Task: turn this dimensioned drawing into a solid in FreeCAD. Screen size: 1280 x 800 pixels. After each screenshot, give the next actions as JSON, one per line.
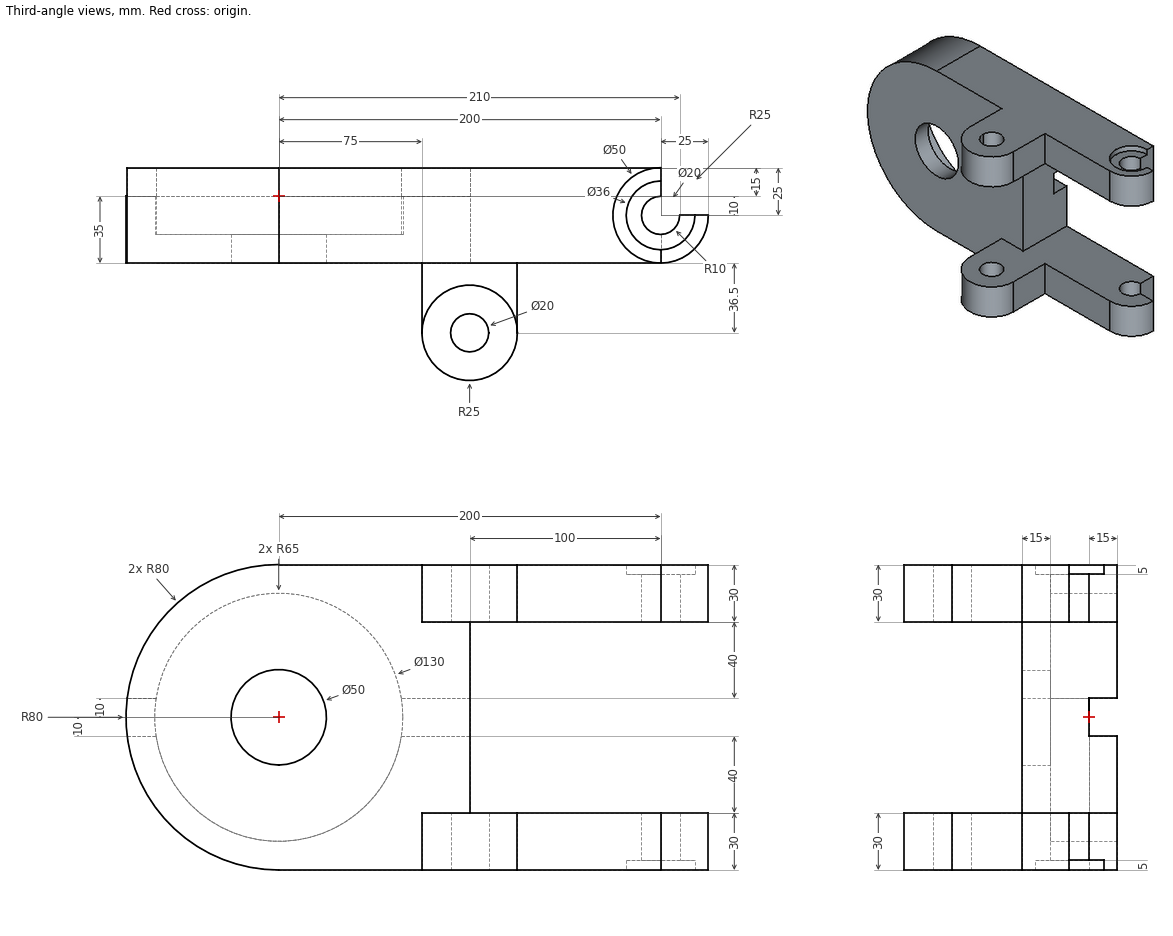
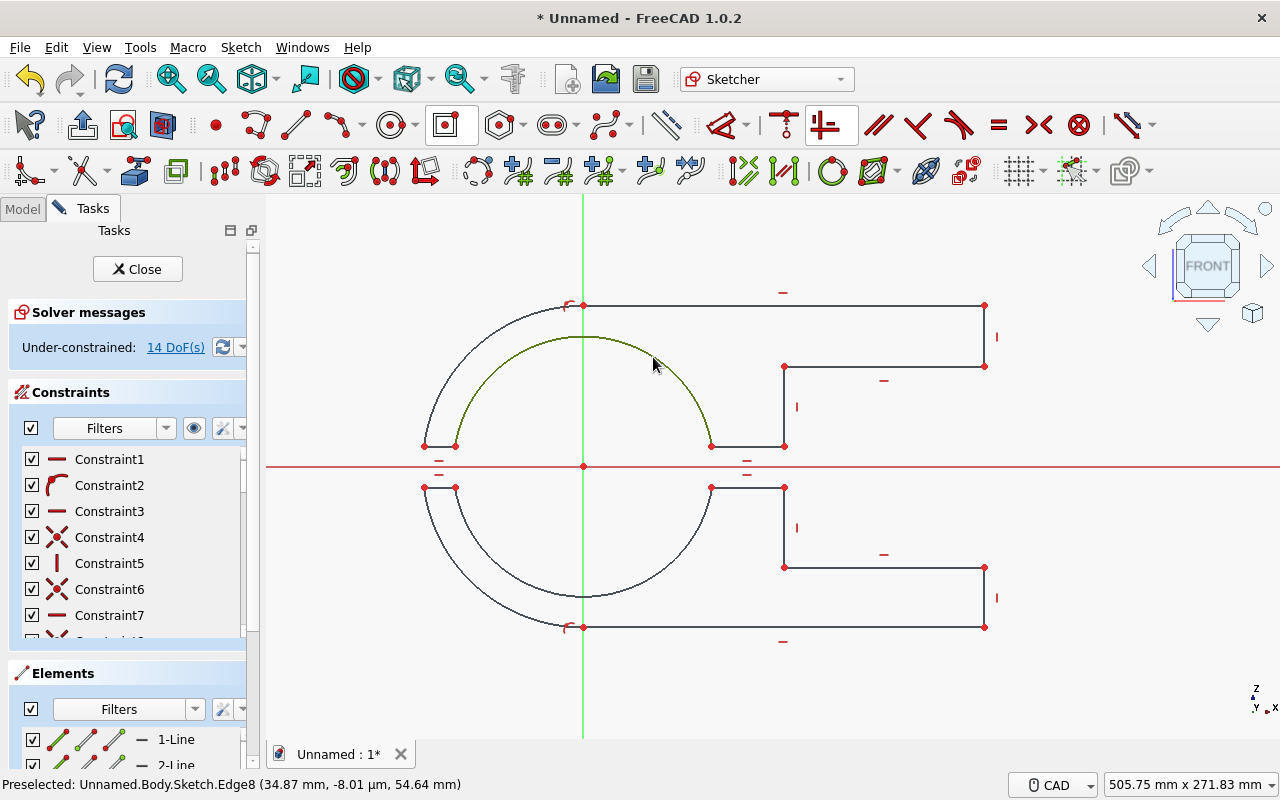
{"action": "left_click", "coordinate": [514, 577]}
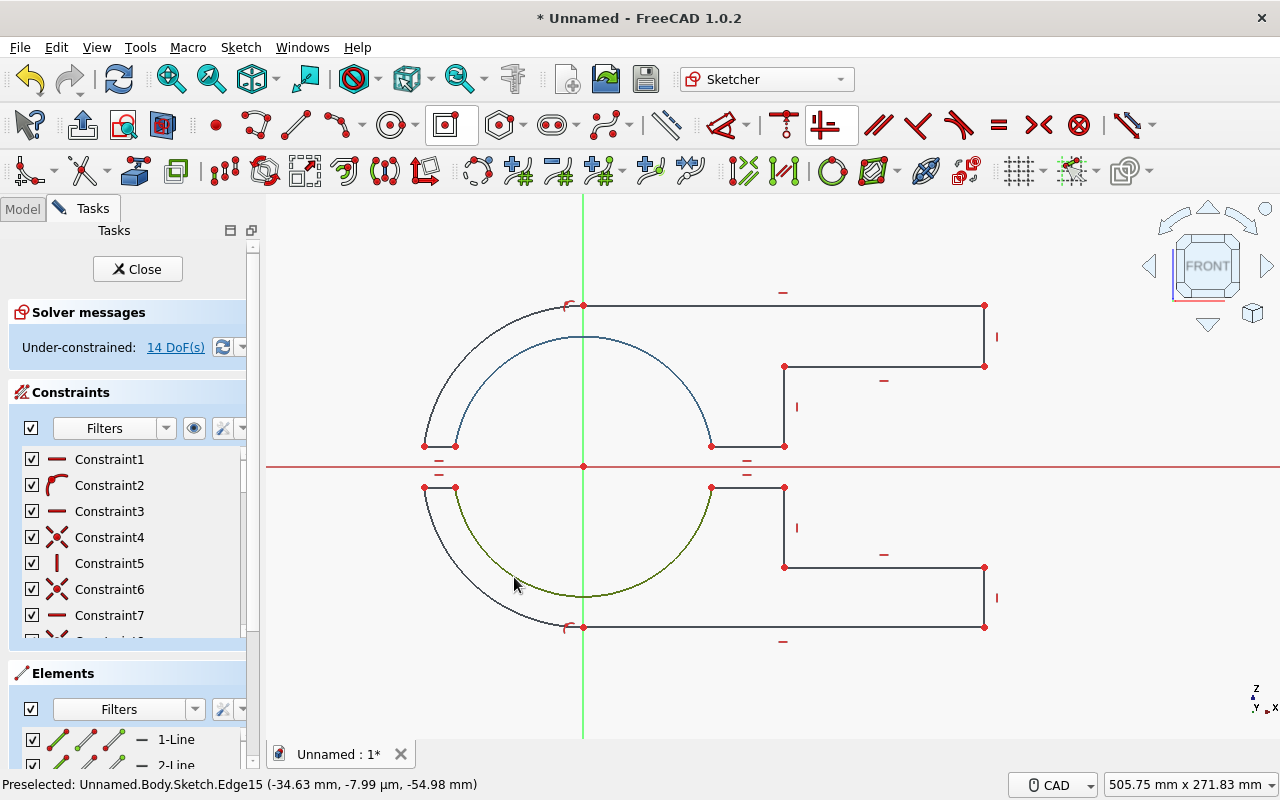
{"action": "left_click", "coordinate": [1000, 126]}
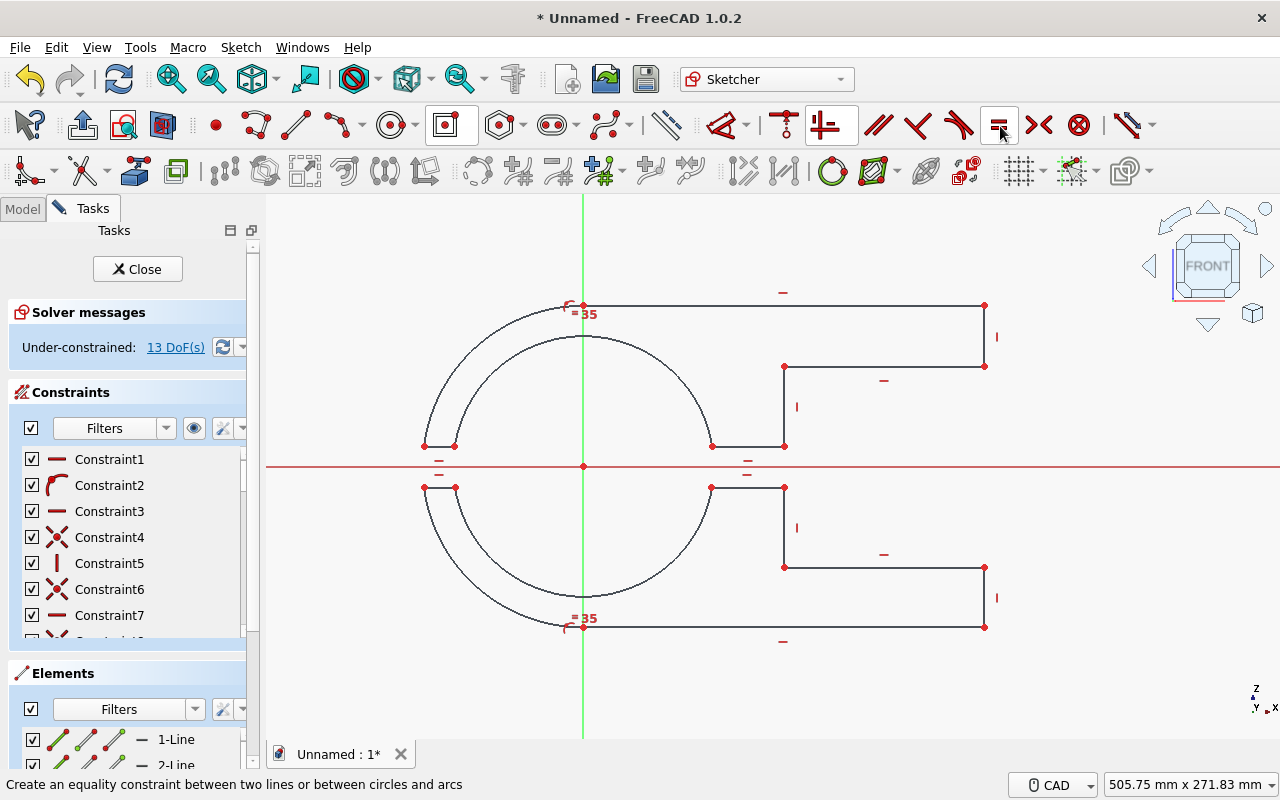
{"action": "left_click", "coordinate": [516, 321]}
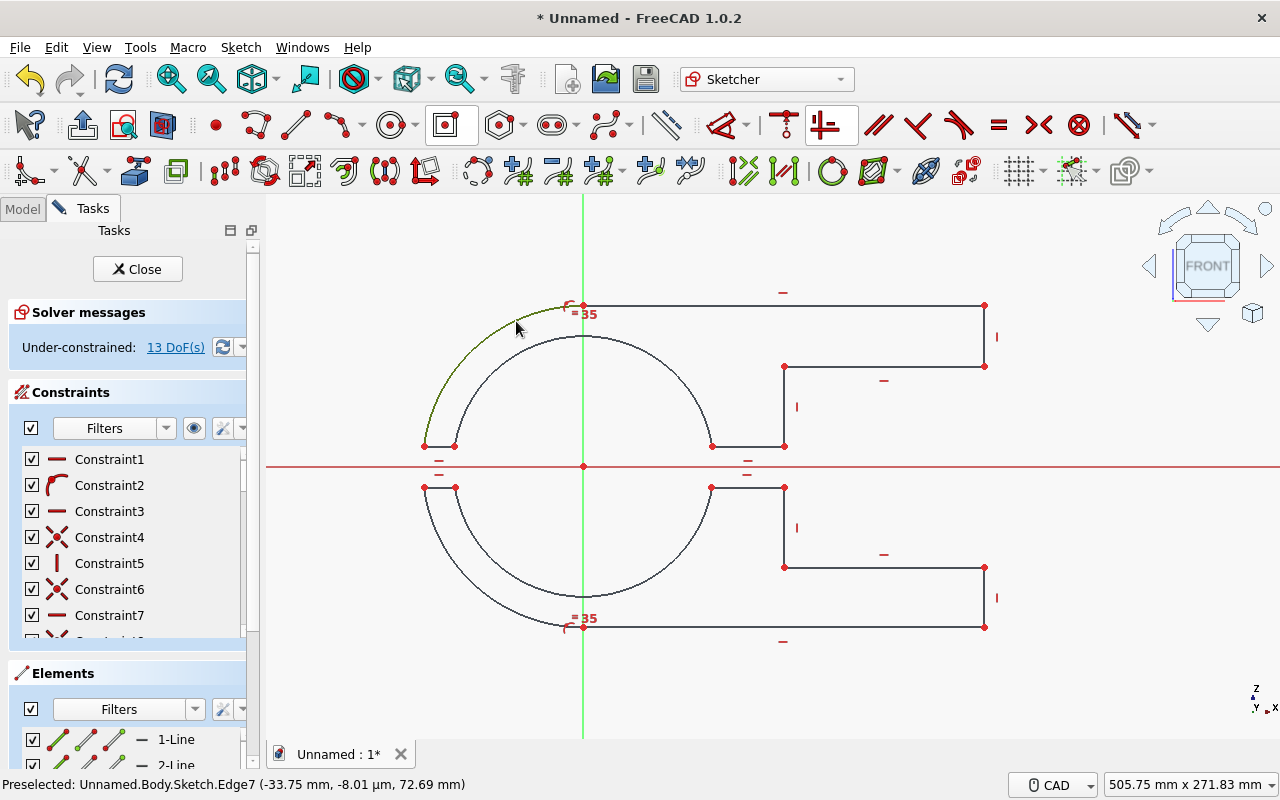
{"action": "left_click", "coordinate": [448, 553]}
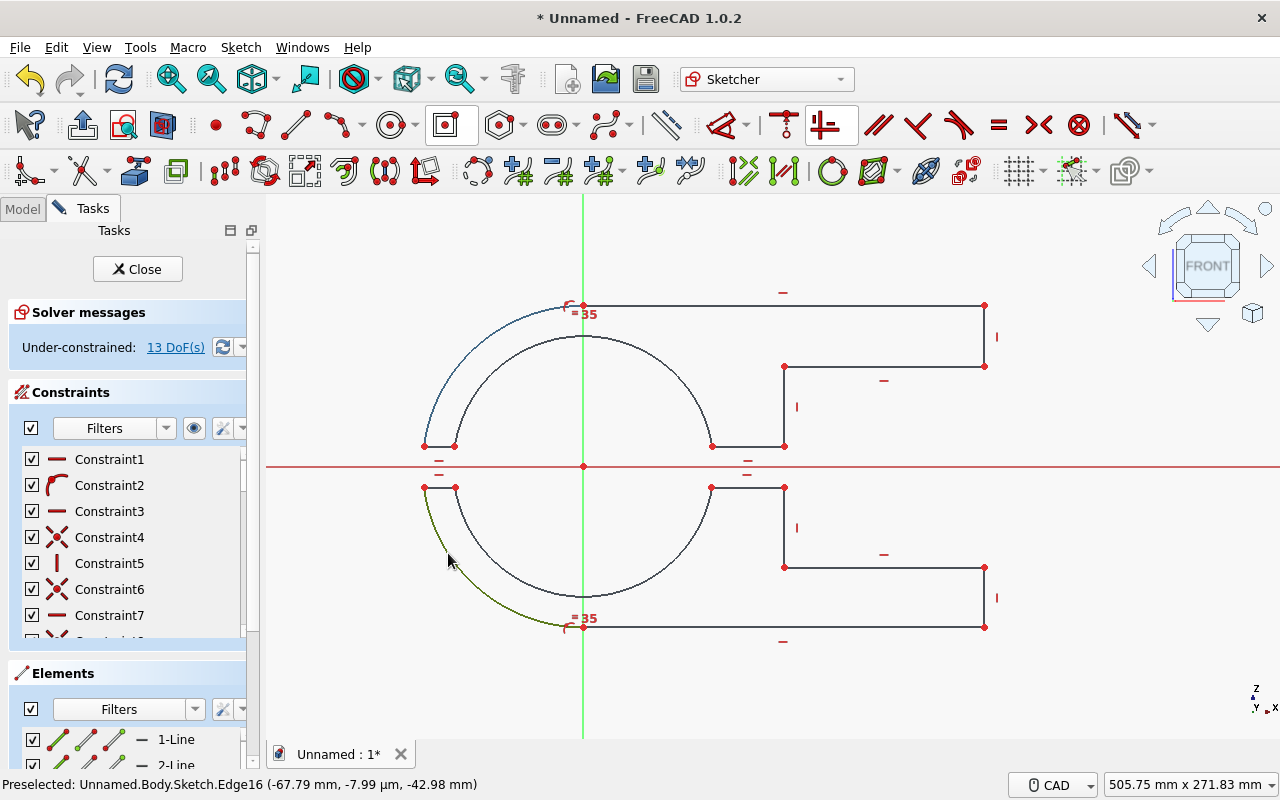
{"action": "key", "text": "e"}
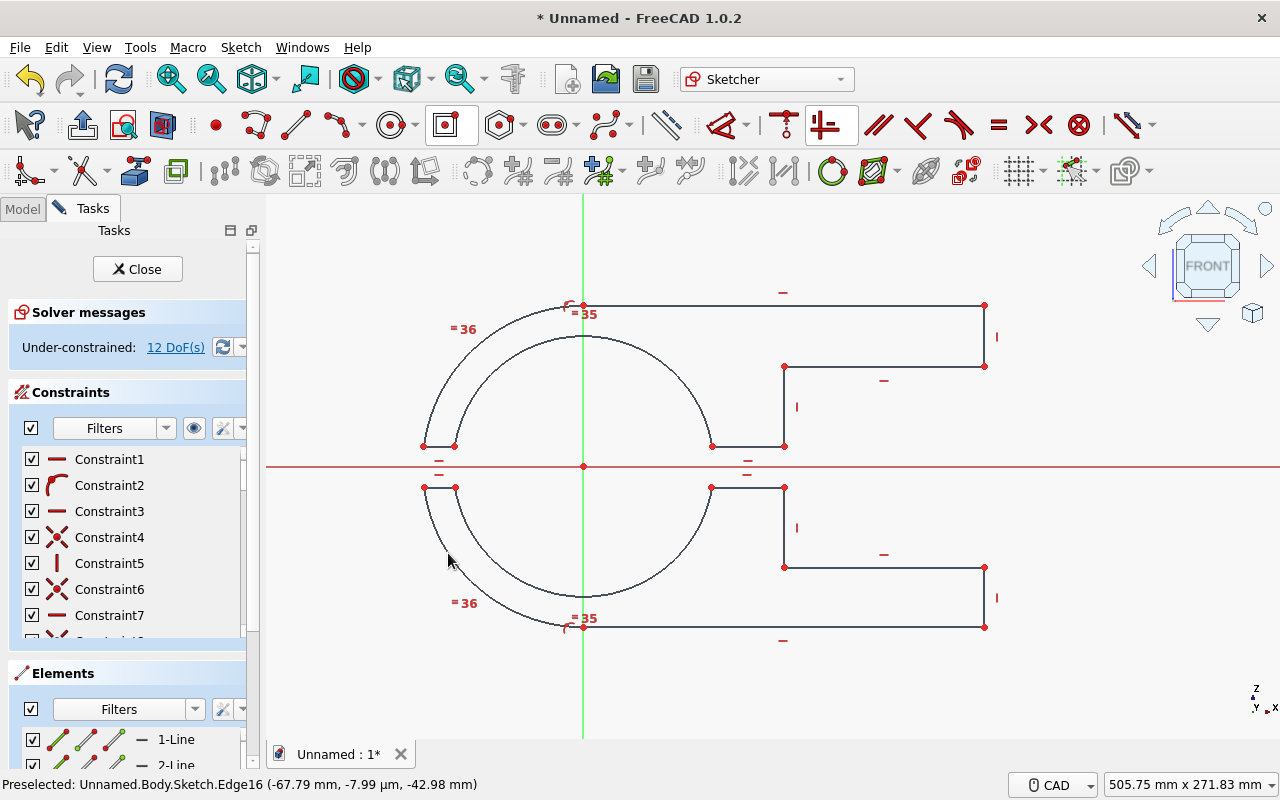
{"action": "left_click", "coordinate": [722, 126]}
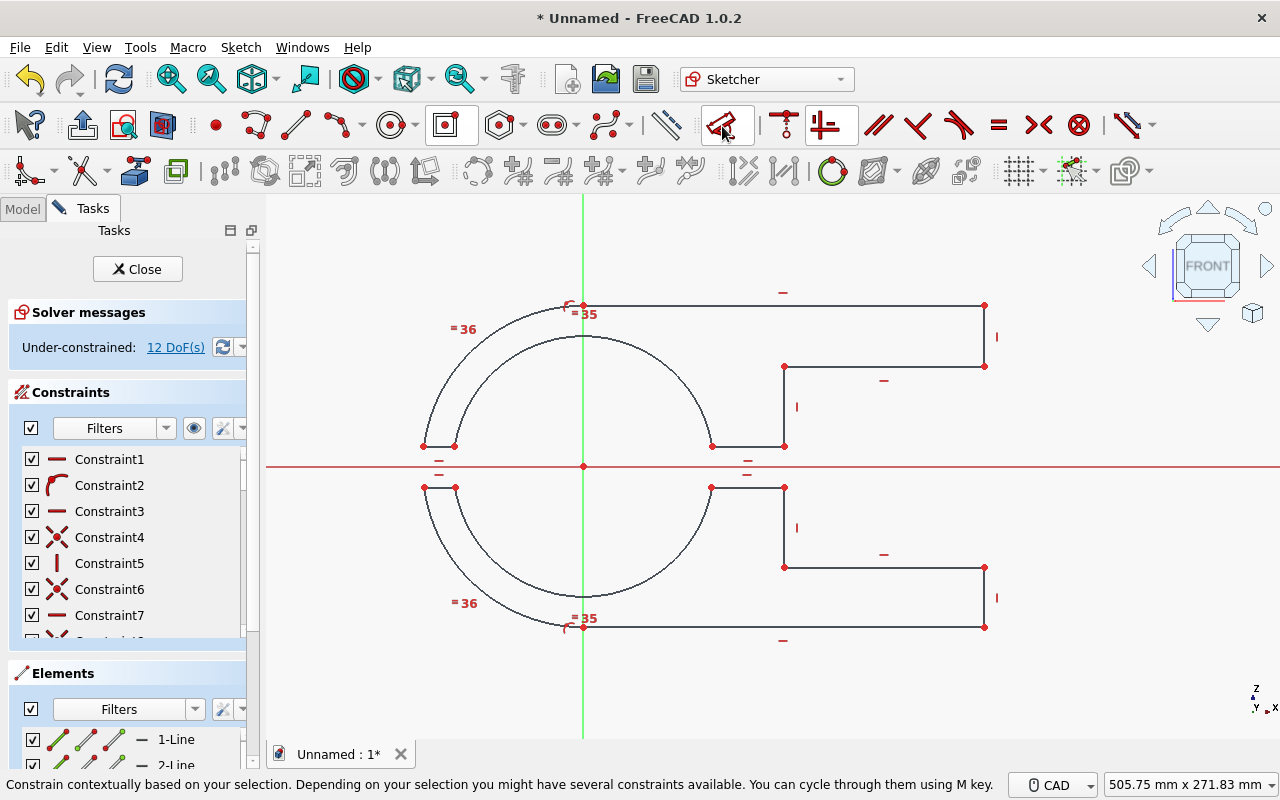
{"action": "left_click", "coordinate": [516, 321]}
{"action": "left_click", "coordinate": [503, 292]}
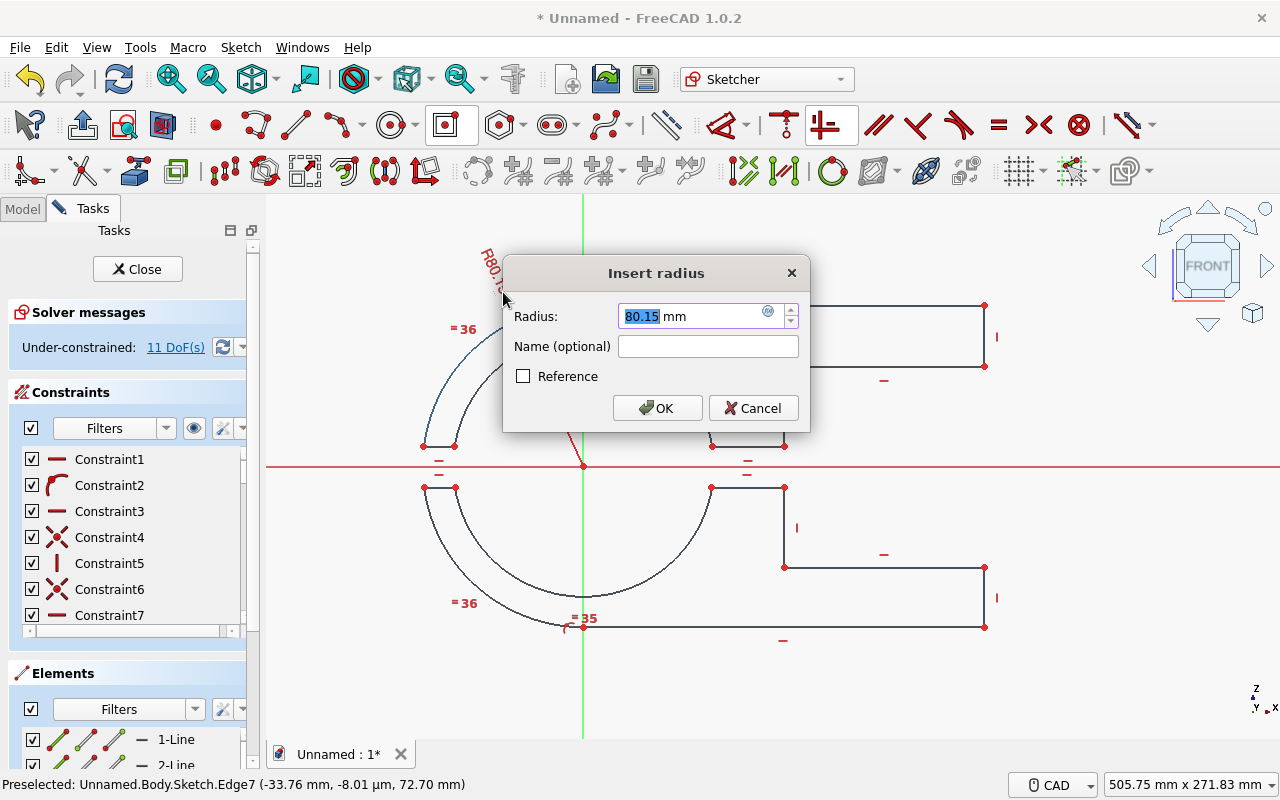
{"action": "type", "text": "80"}
{"action": "key", "text": "Return"}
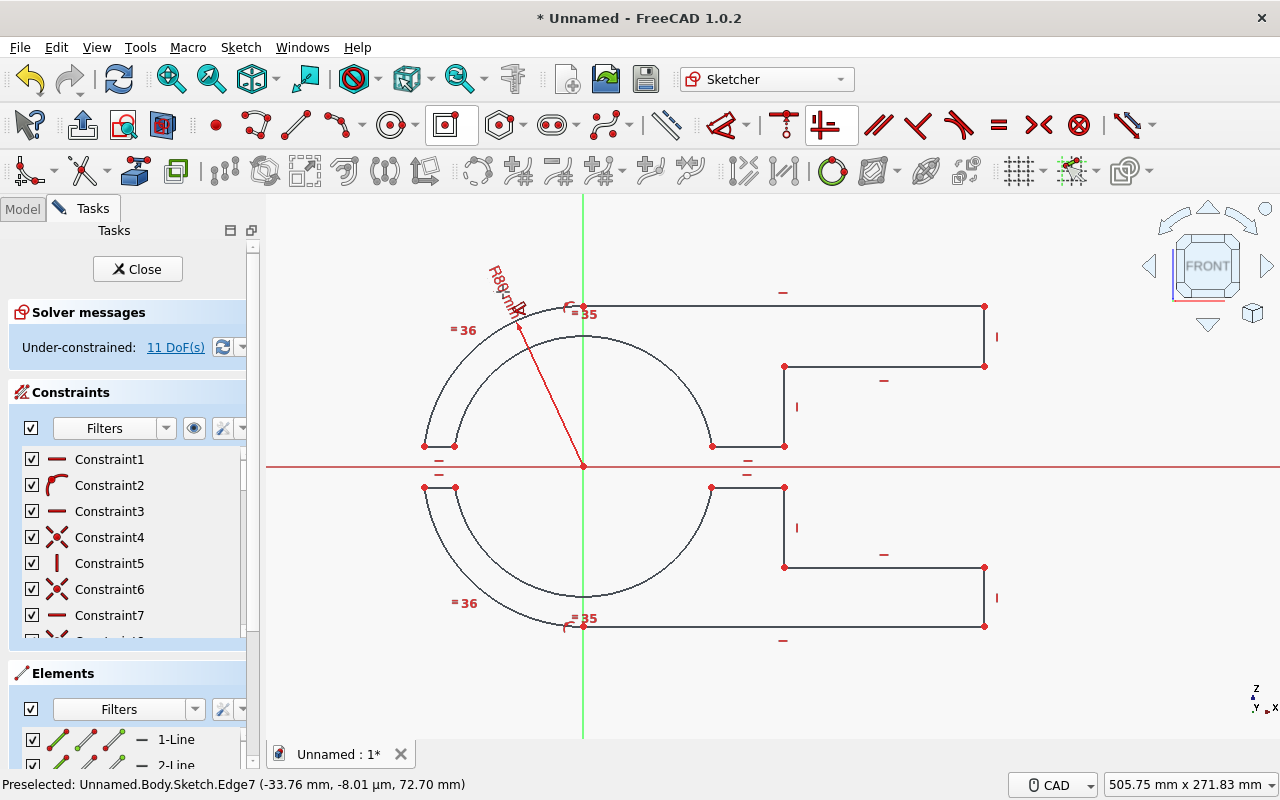
{"action": "left_click", "coordinate": [654, 357]}
{"action": "left_click", "coordinate": [671, 330]}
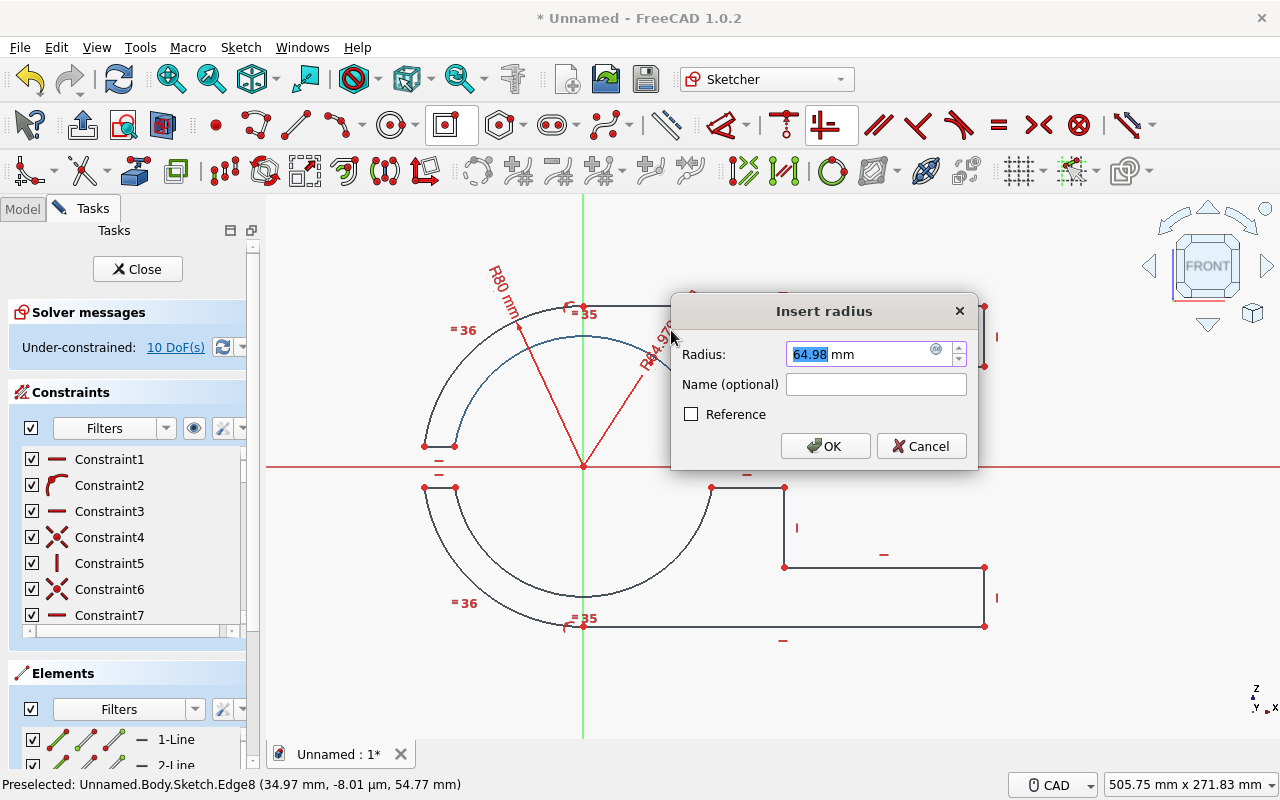
{"action": "type", "text": "65"}
{"action": "key", "text": "Return"}